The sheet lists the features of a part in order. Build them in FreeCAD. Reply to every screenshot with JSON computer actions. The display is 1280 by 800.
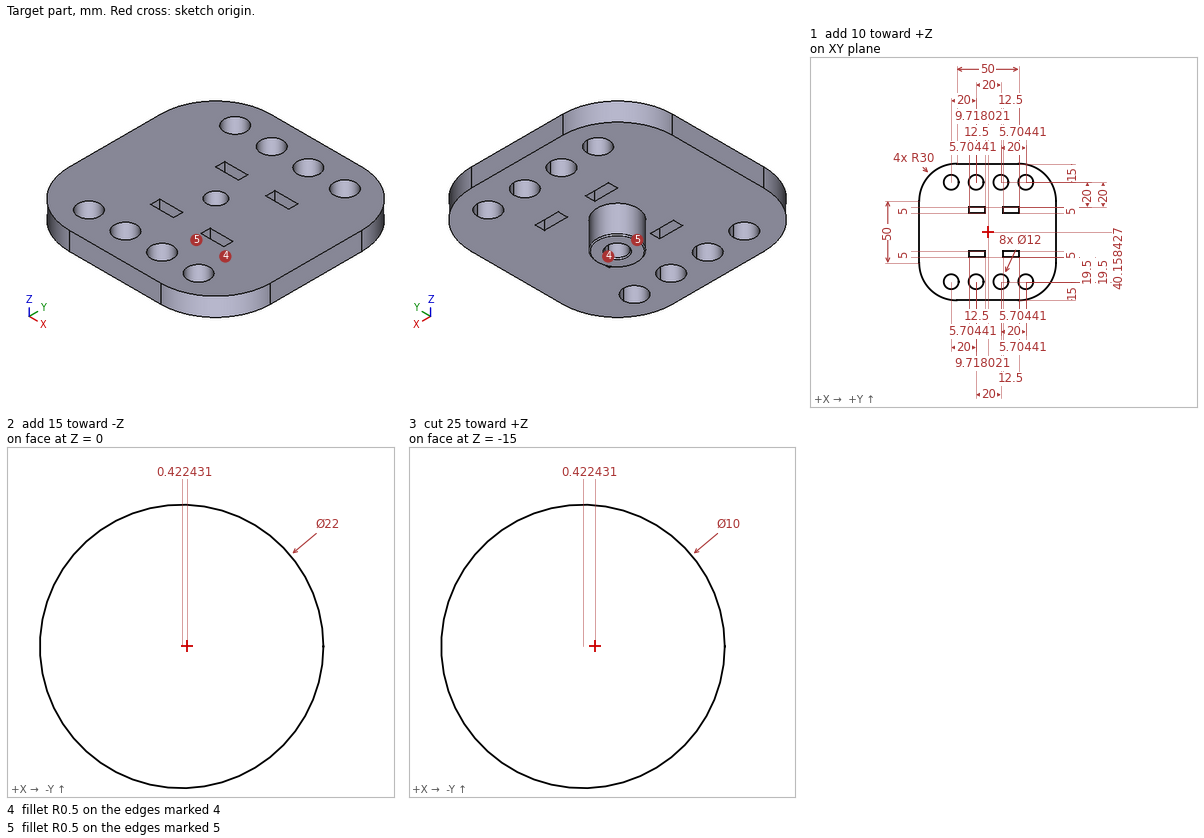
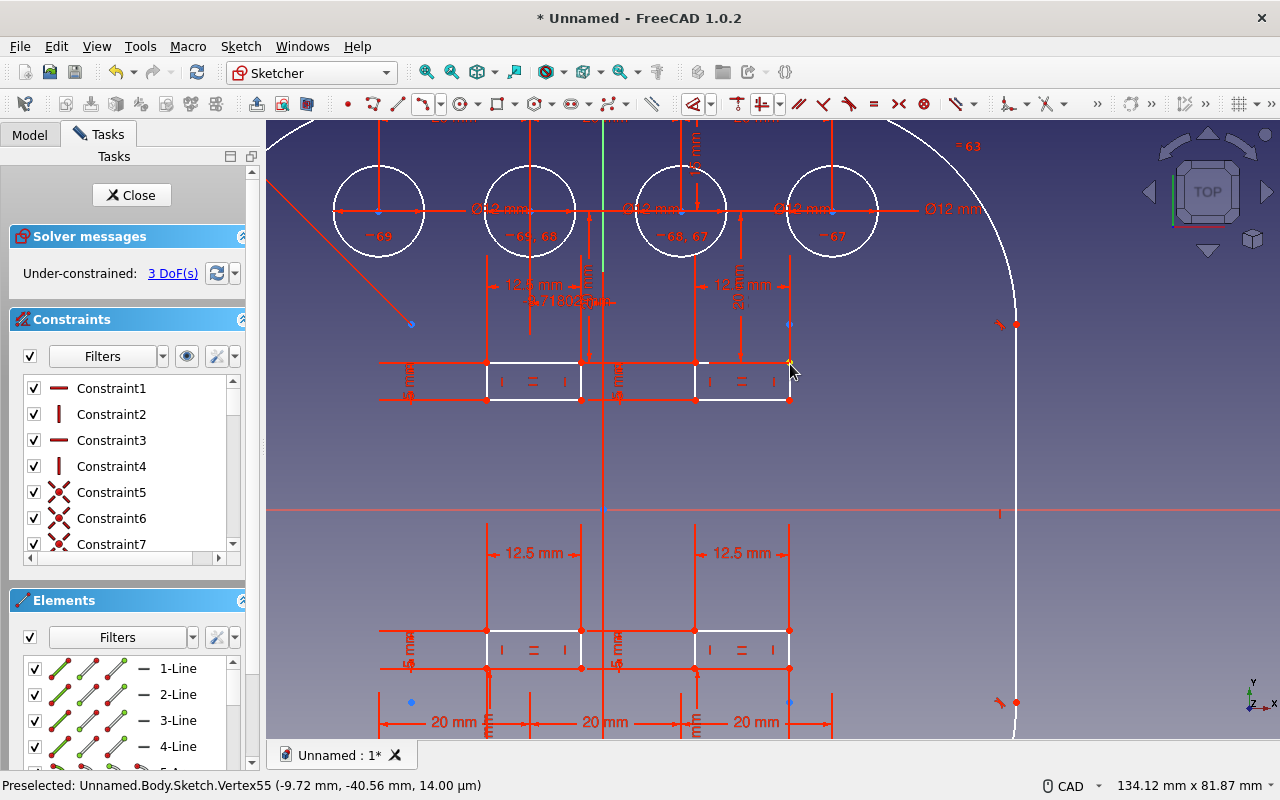
{"action": "left_click", "coordinate": [790, 363]}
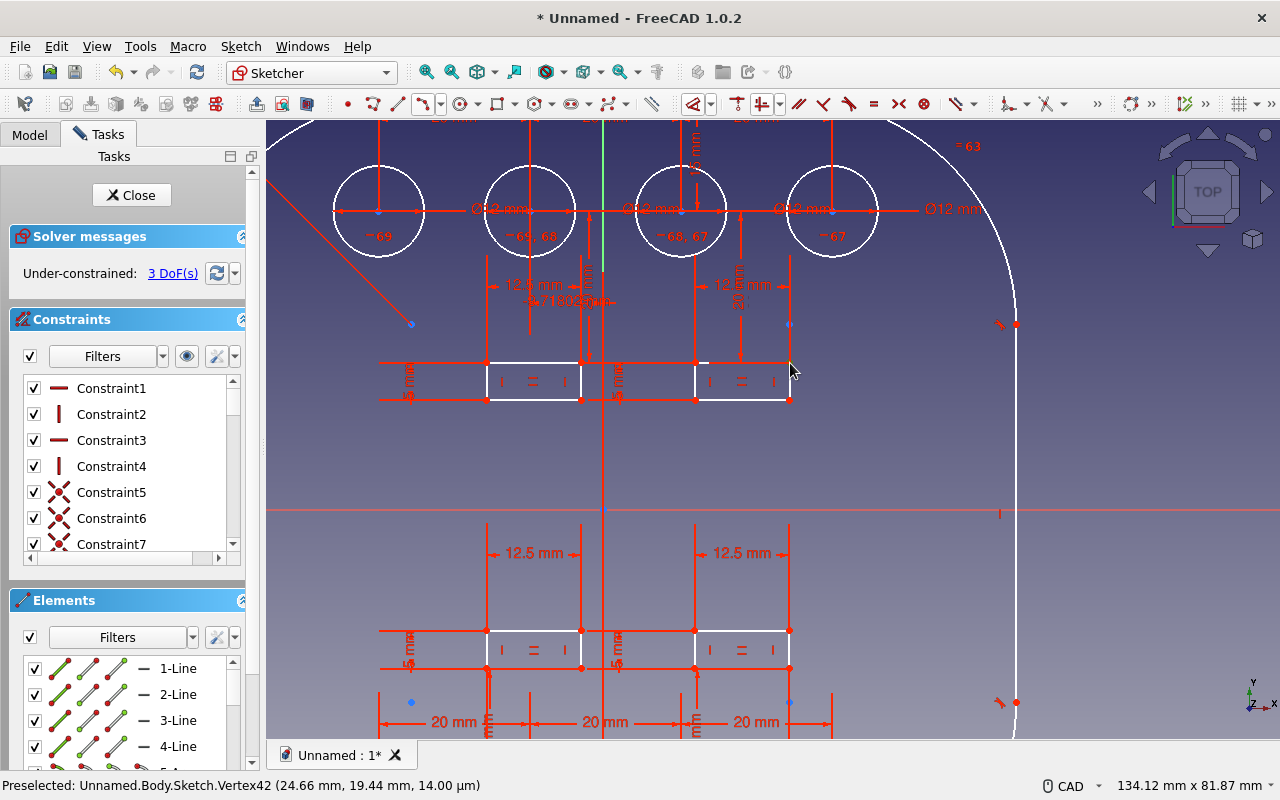
{"action": "left_click", "coordinate": [832, 211]}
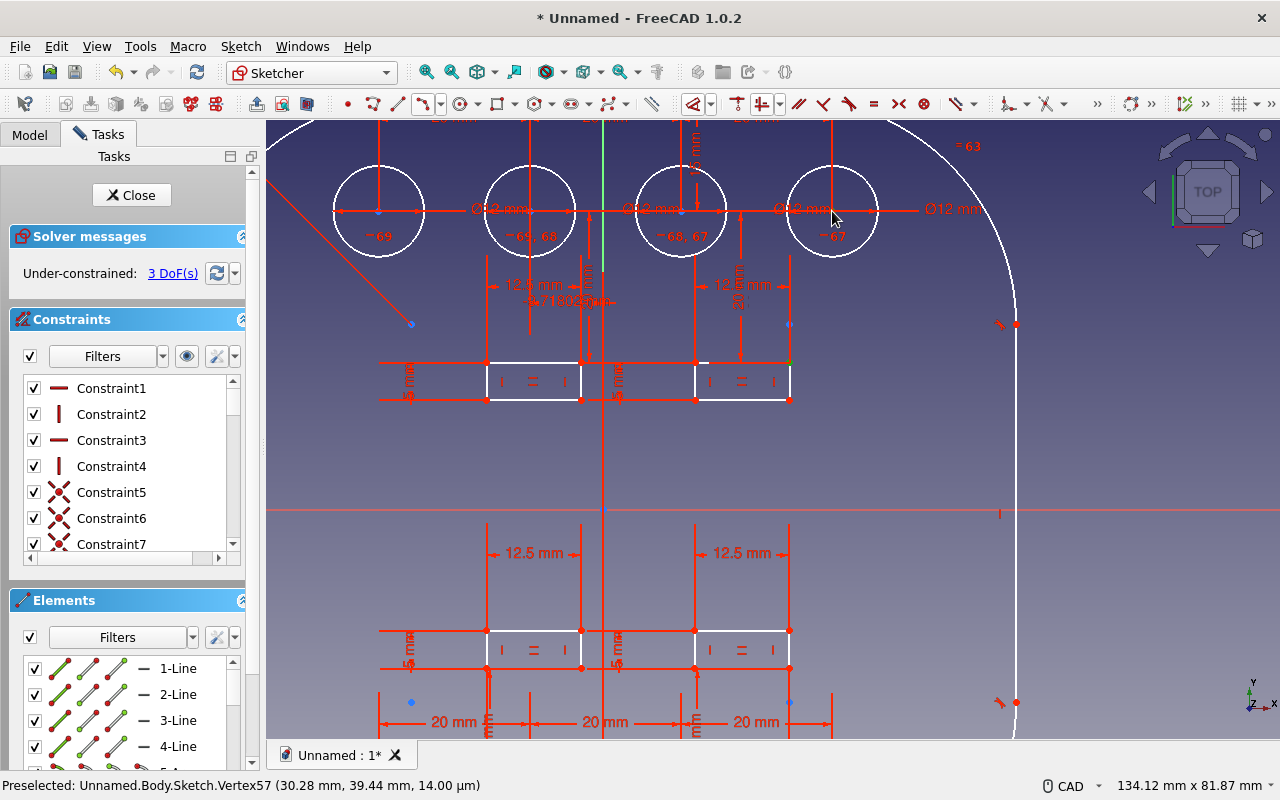
{"action": "left_click", "coordinate": [710, 104]}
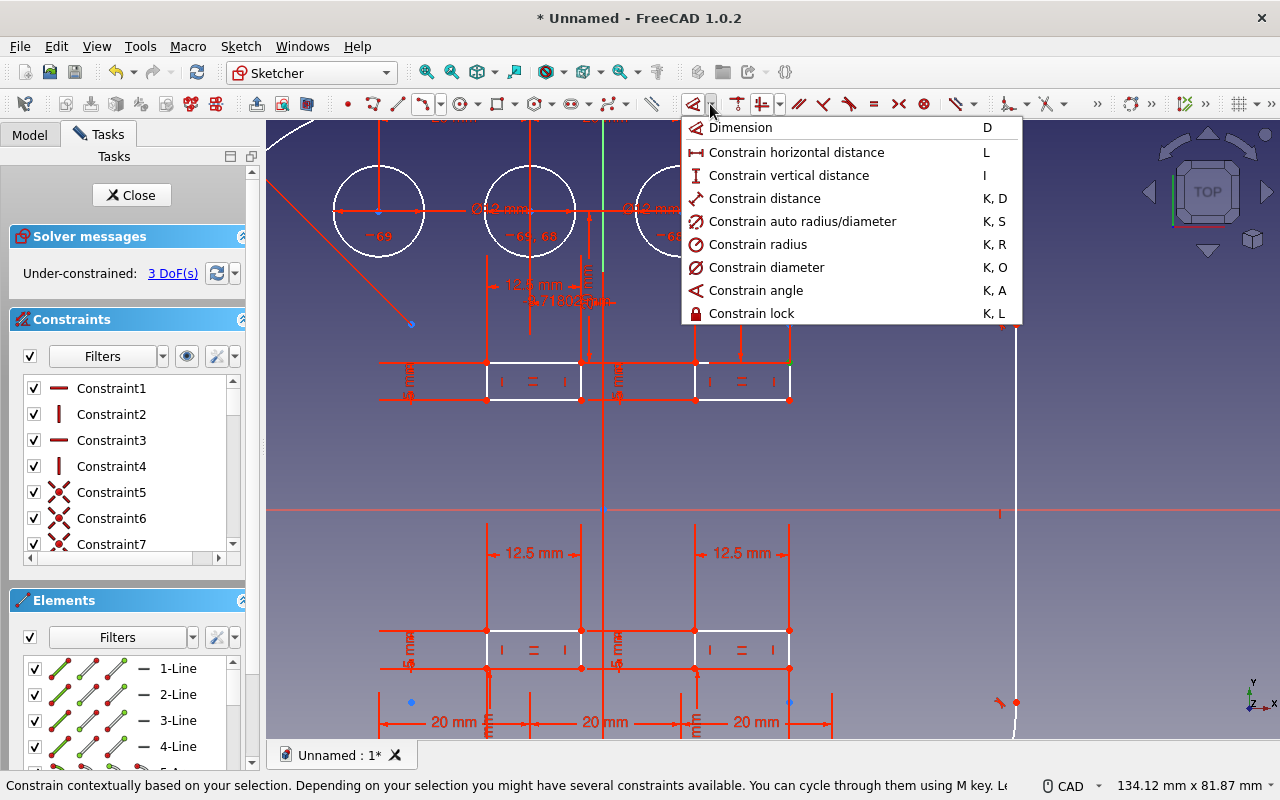
{"action": "left_click", "coordinate": [852, 152]}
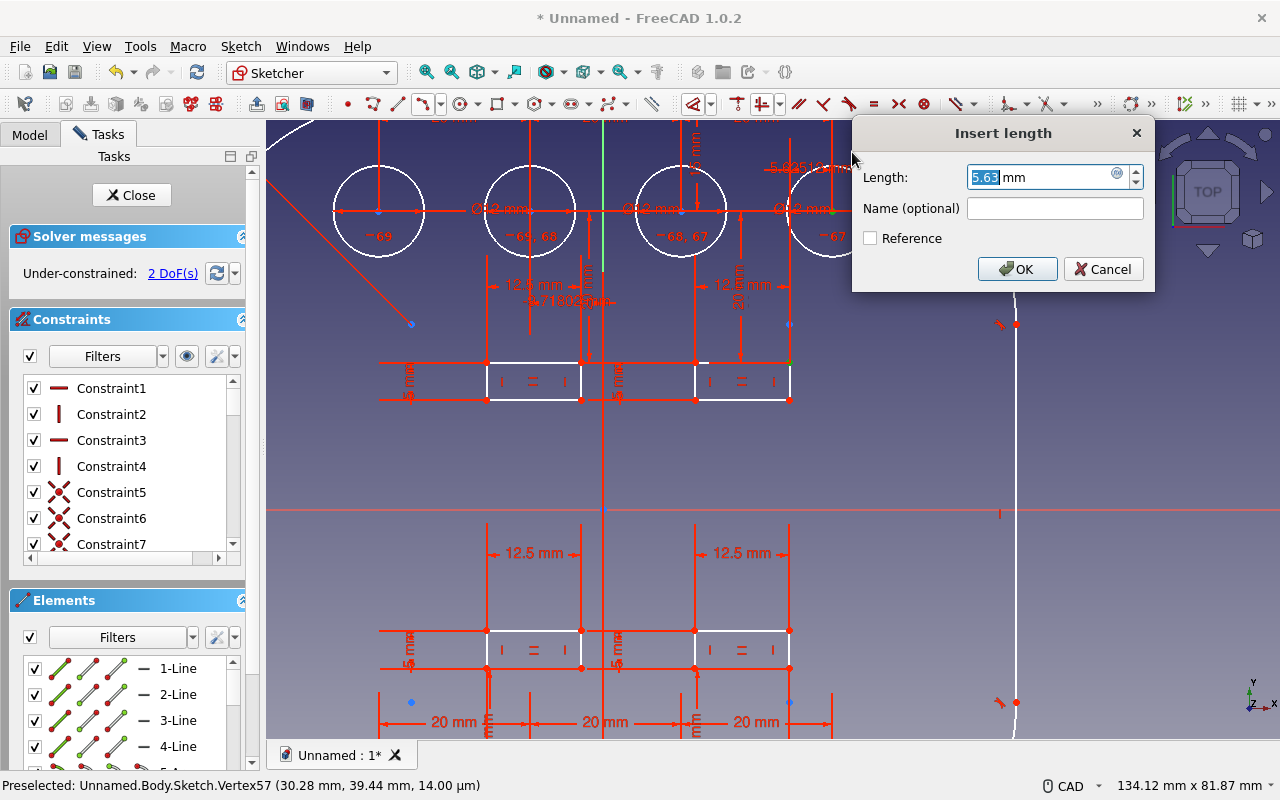
{"action": "type", "text": "5.70441"}
{"action": "key", "text": "Return"}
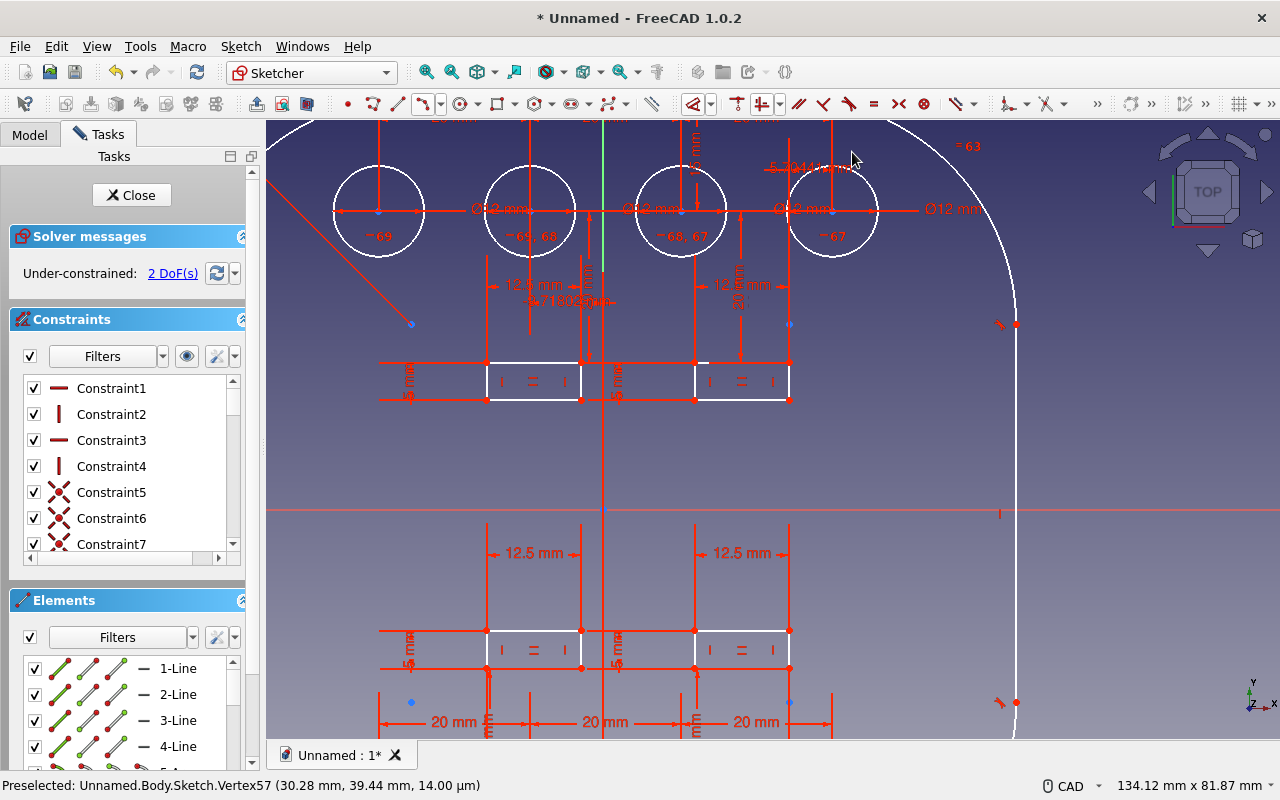
{"action": "left_click", "coordinate": [487, 363]}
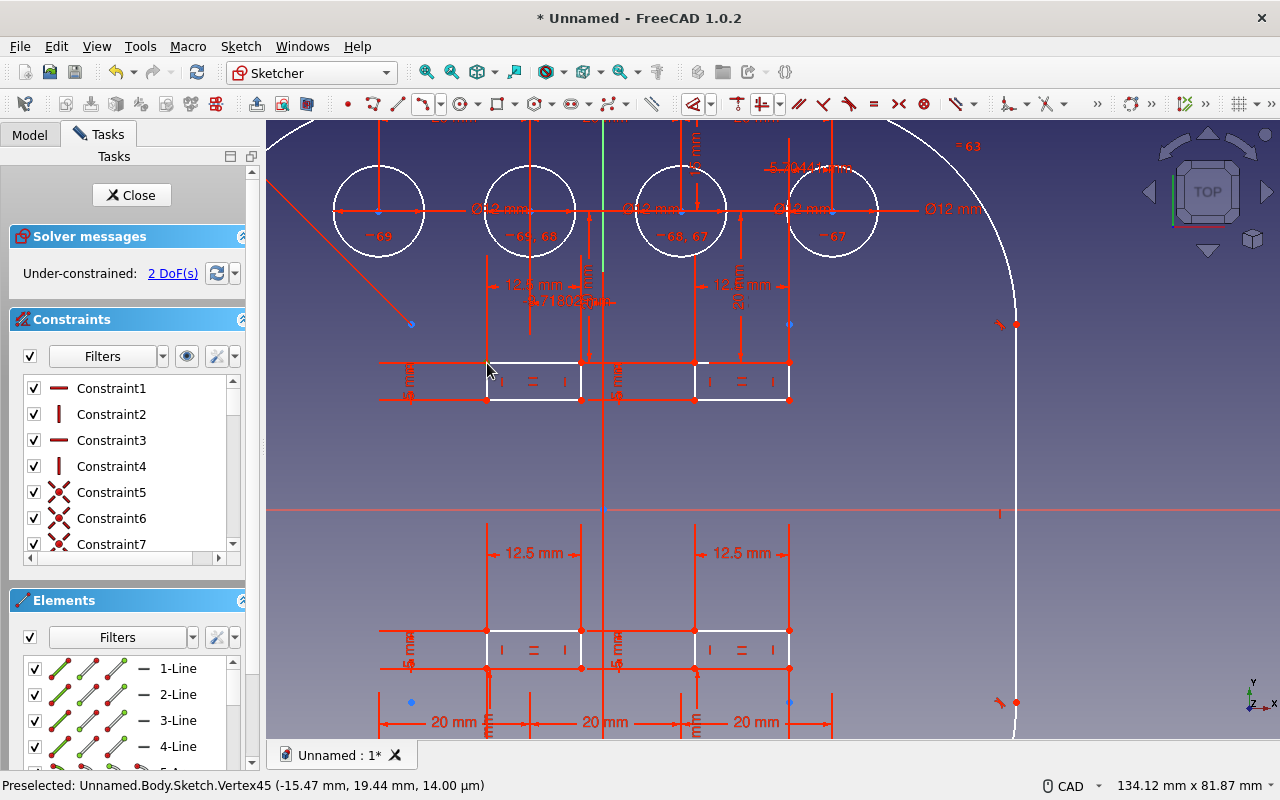
{"action": "left_click", "coordinate": [530, 211]}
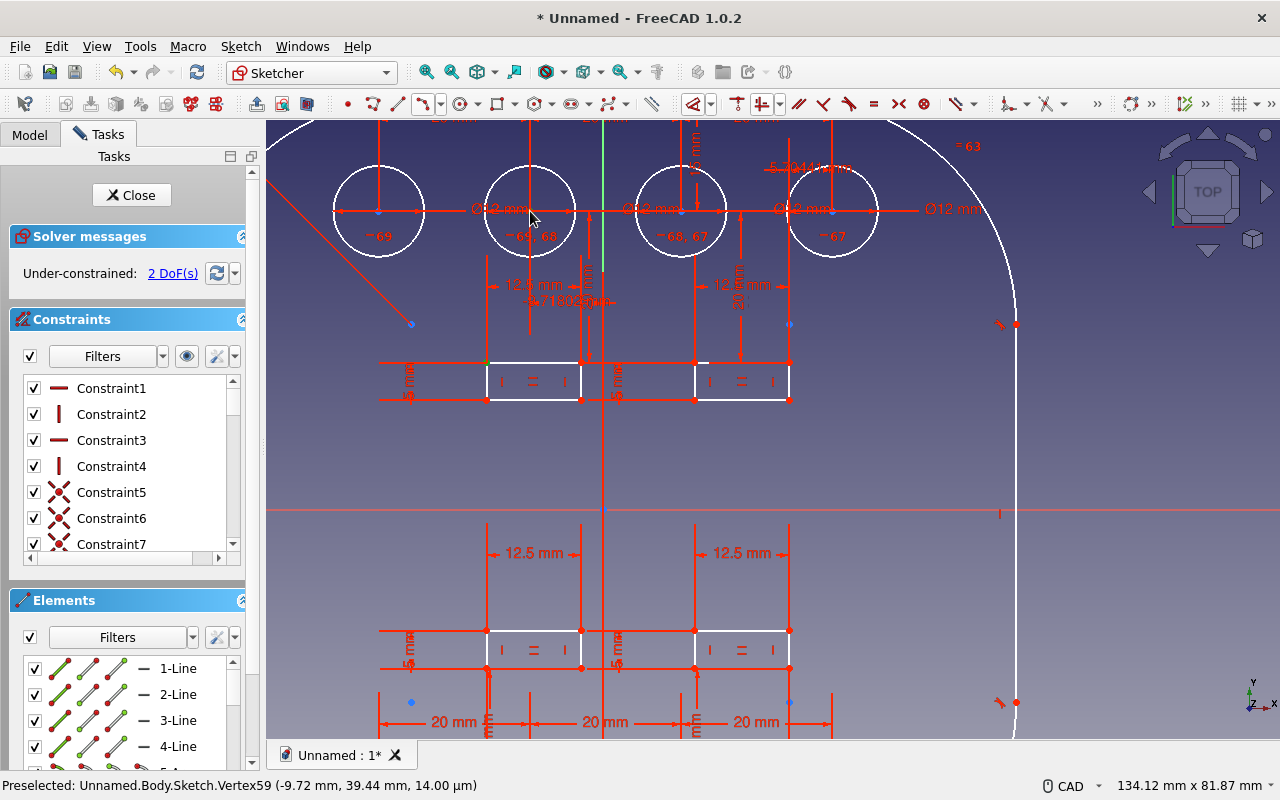
{"action": "key", "text": "l"}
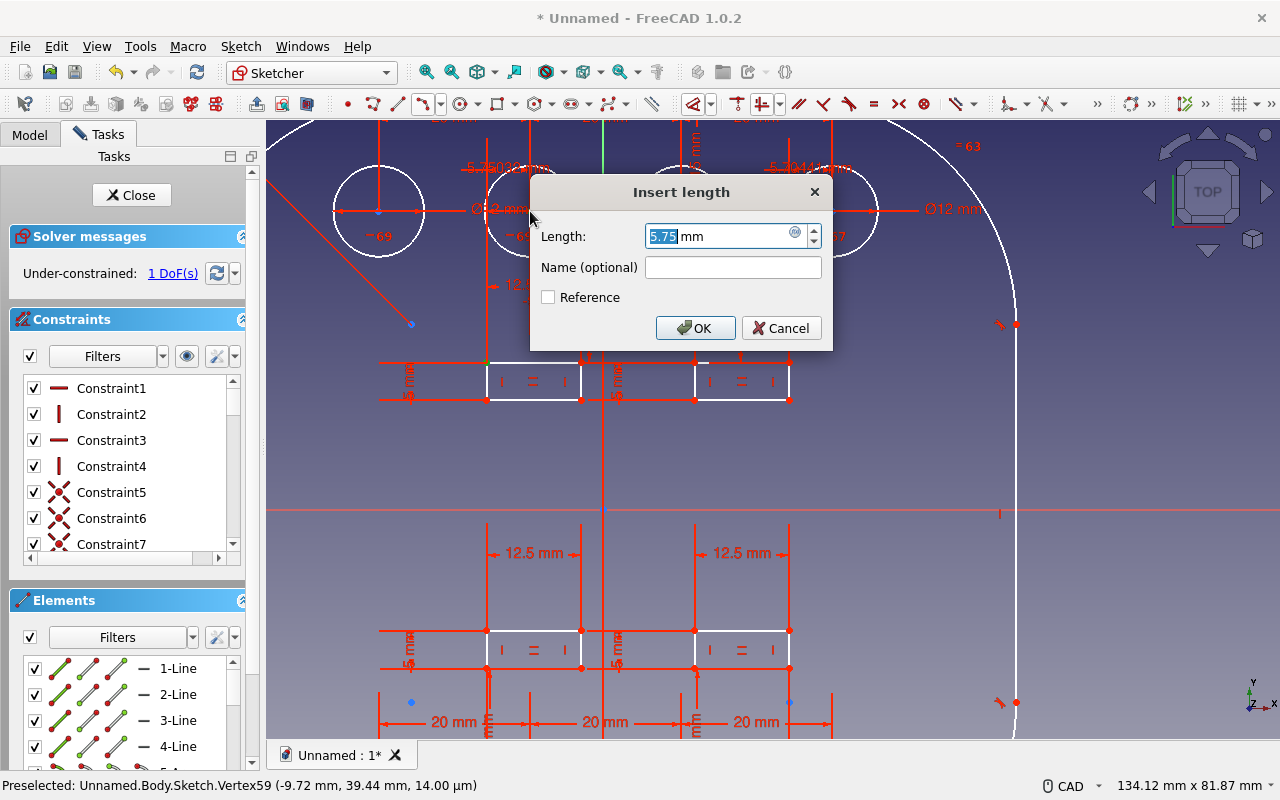
{"action": "type", "text": "5.70441"}
{"action": "key", "text": "Return"}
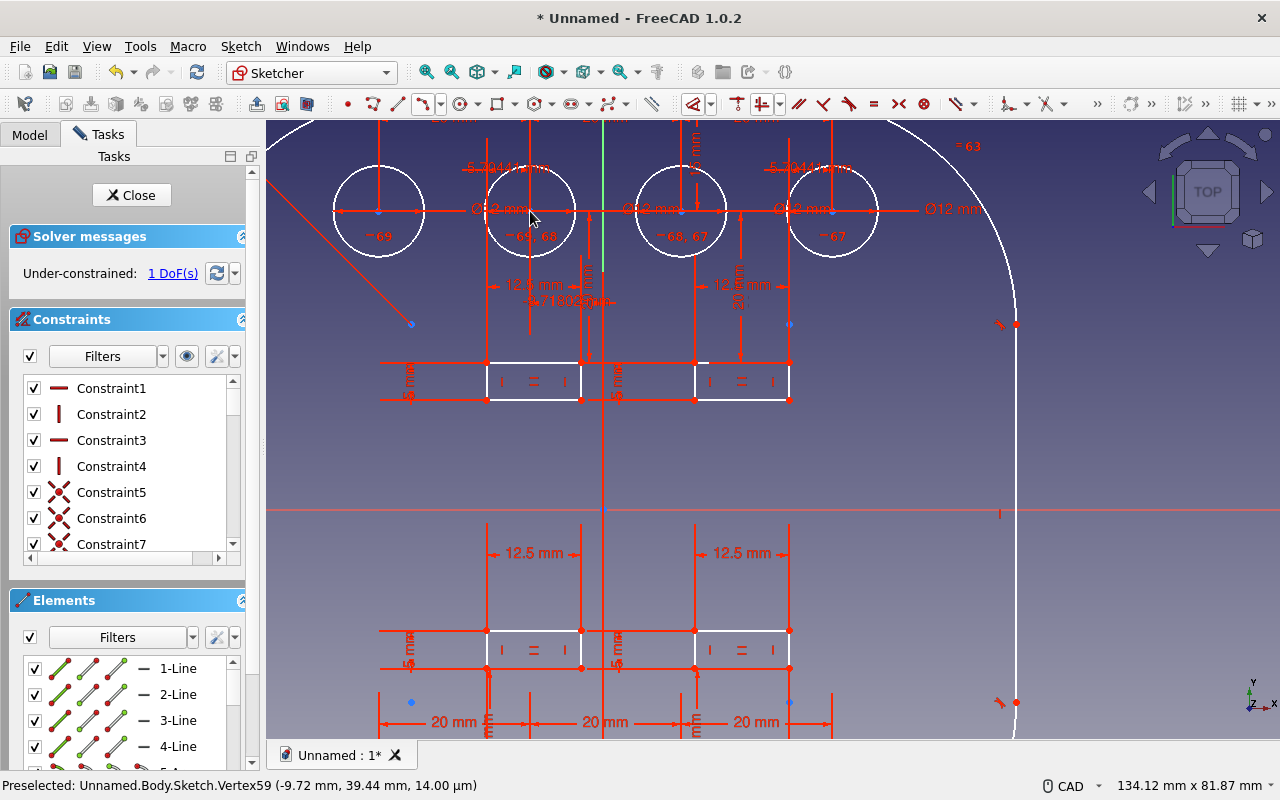
{"action": "scroll", "coordinate": [790, 363], "scroll_direction": "down", "scroll_amount": 4}